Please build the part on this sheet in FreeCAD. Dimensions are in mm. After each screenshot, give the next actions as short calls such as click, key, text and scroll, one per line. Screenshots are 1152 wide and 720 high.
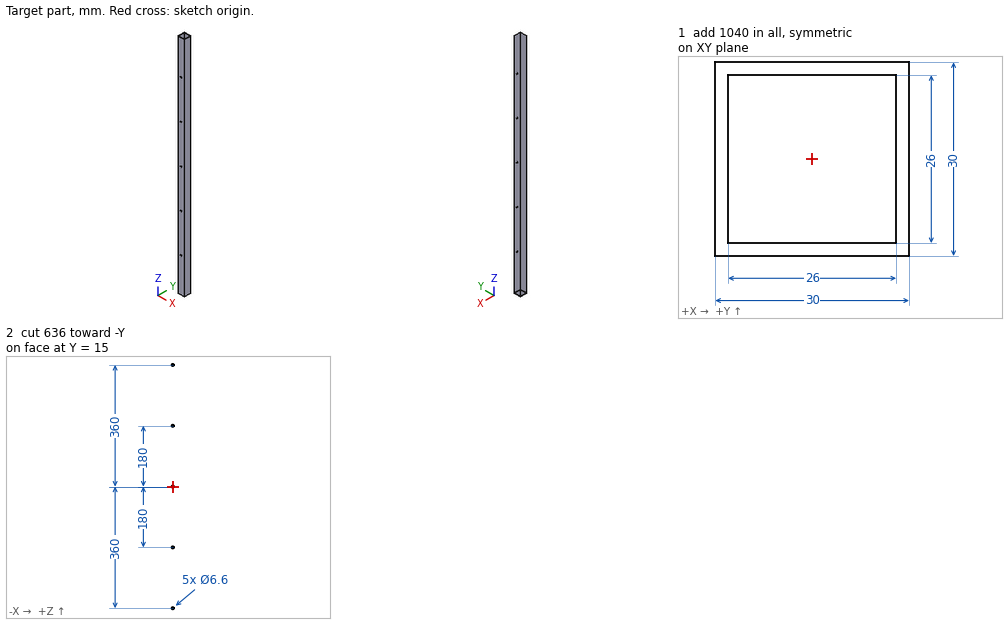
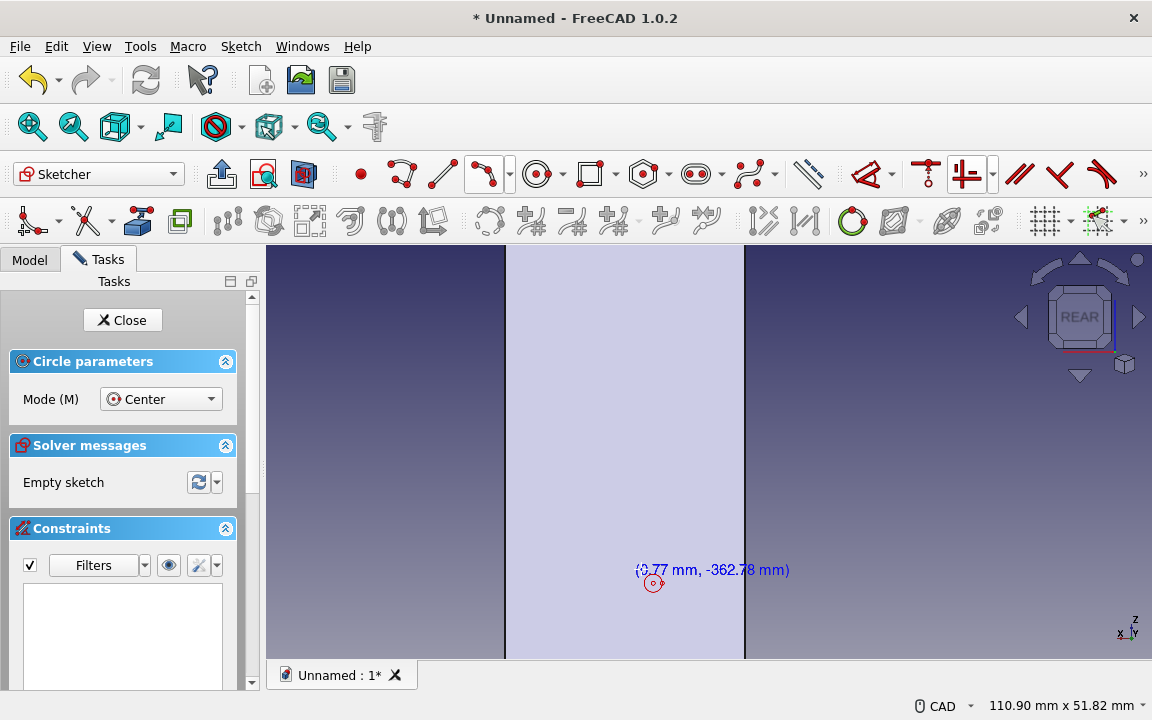
scroll(641, 597, down, 15)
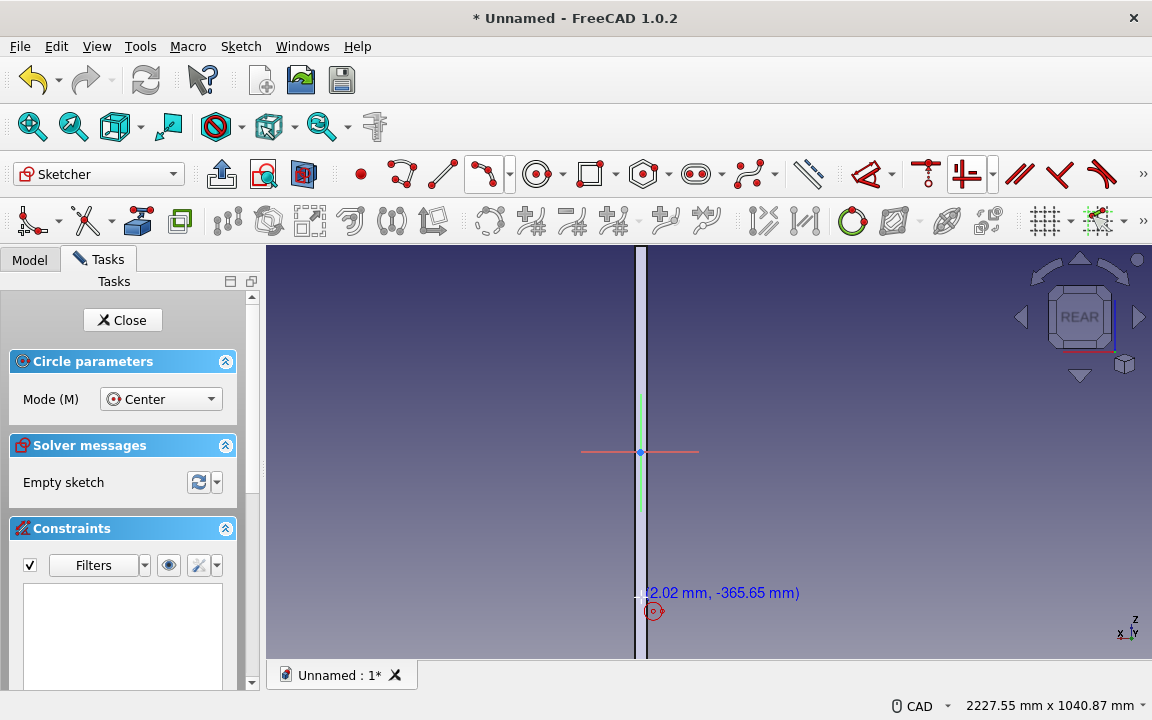
click(641, 596)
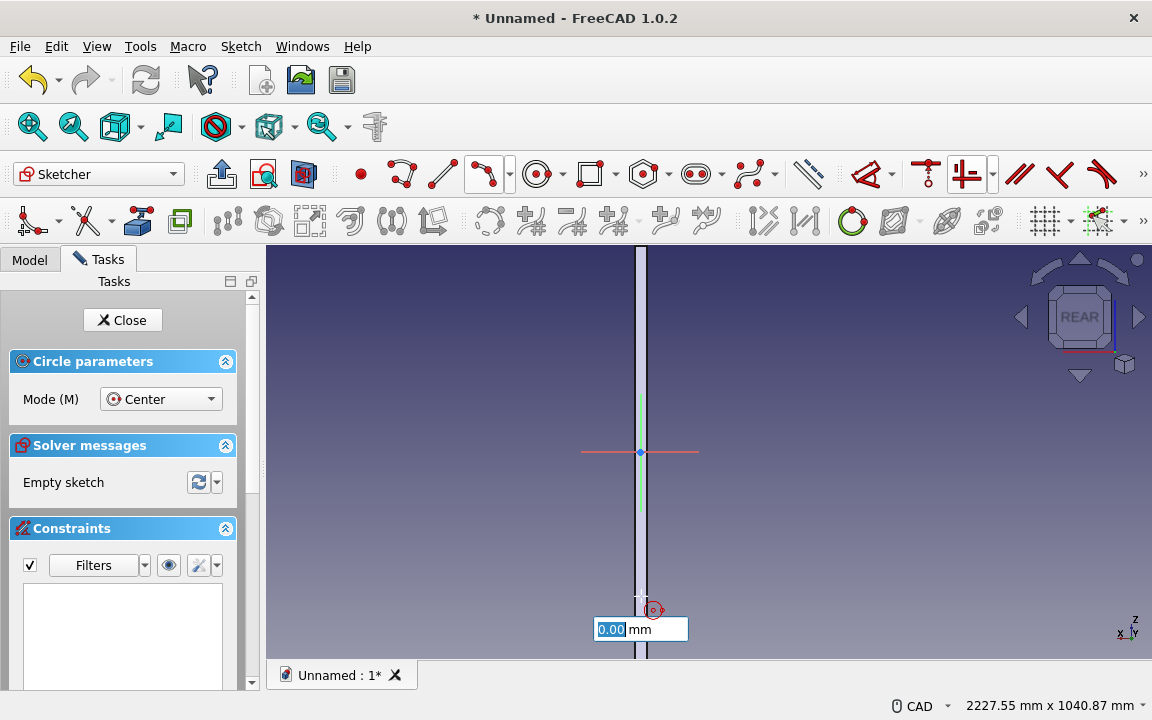
scroll(642, 595, up, 13)
move(634, 587)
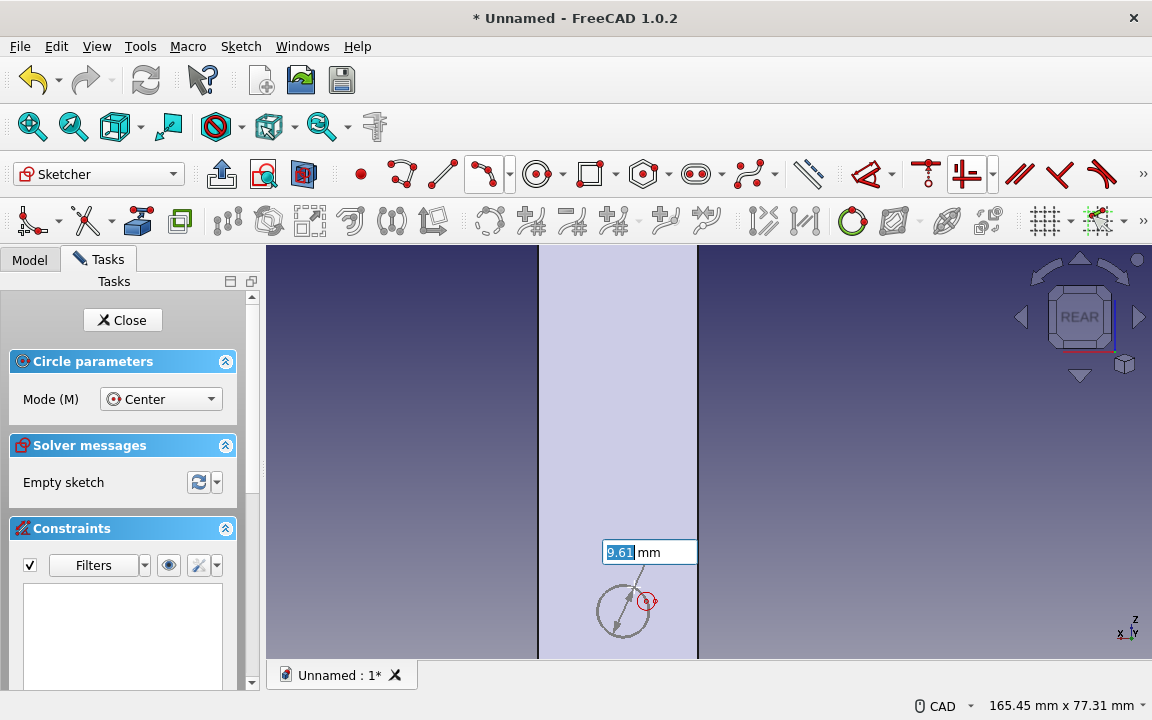
text(6.6)
key(Return)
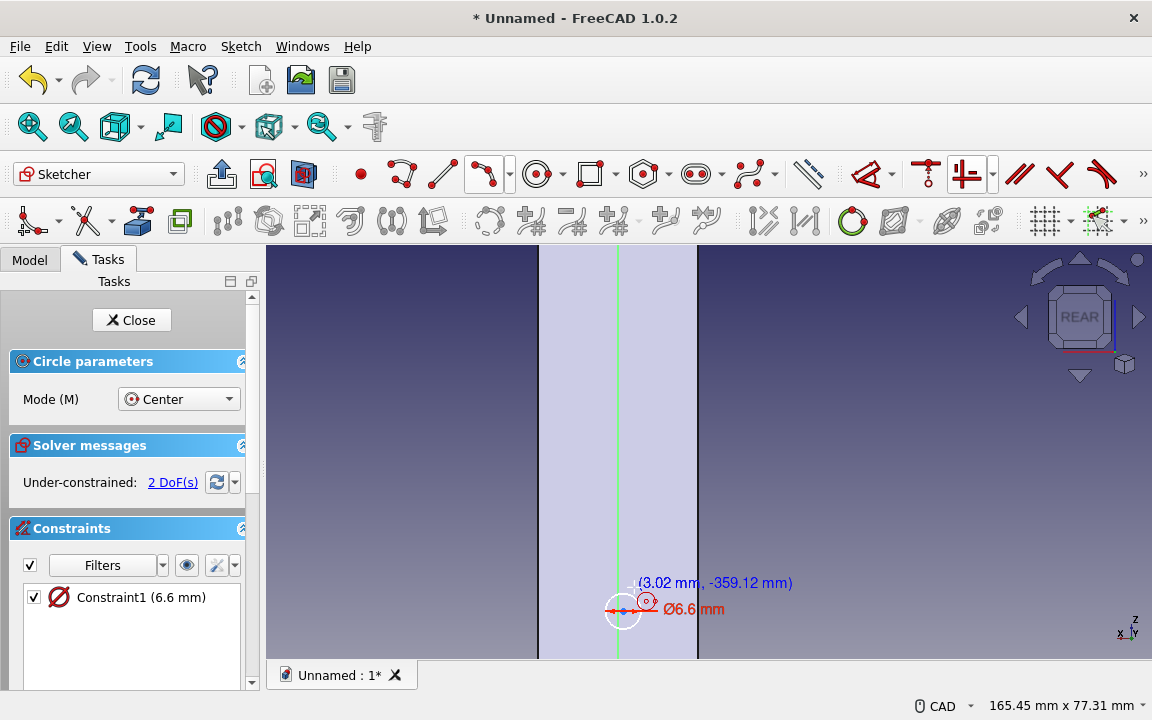
scroll(642, 568, down, 14)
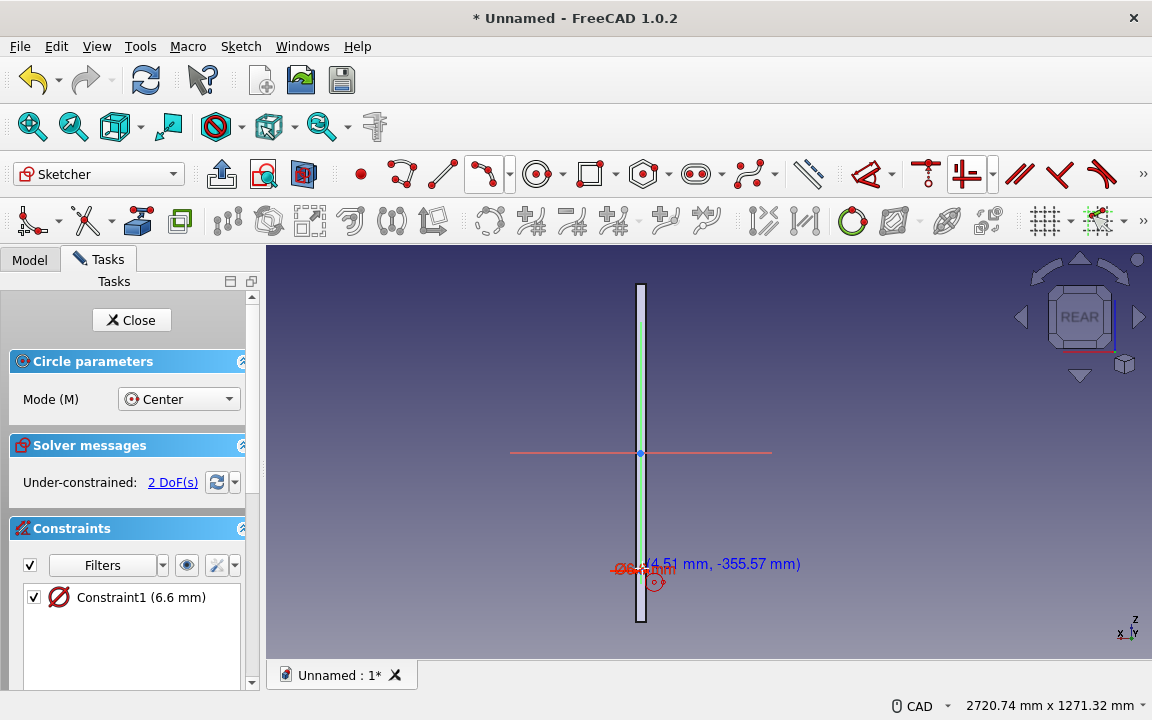
scroll(641, 512, up, 16)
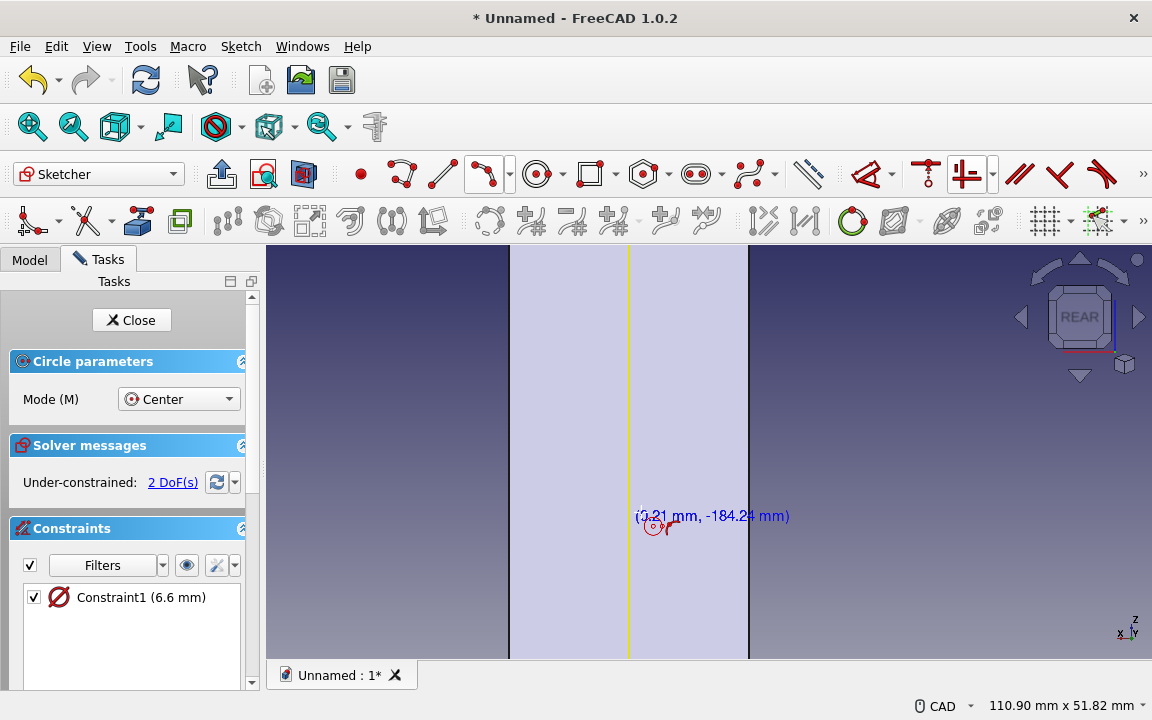
scroll(641, 525, down, 15)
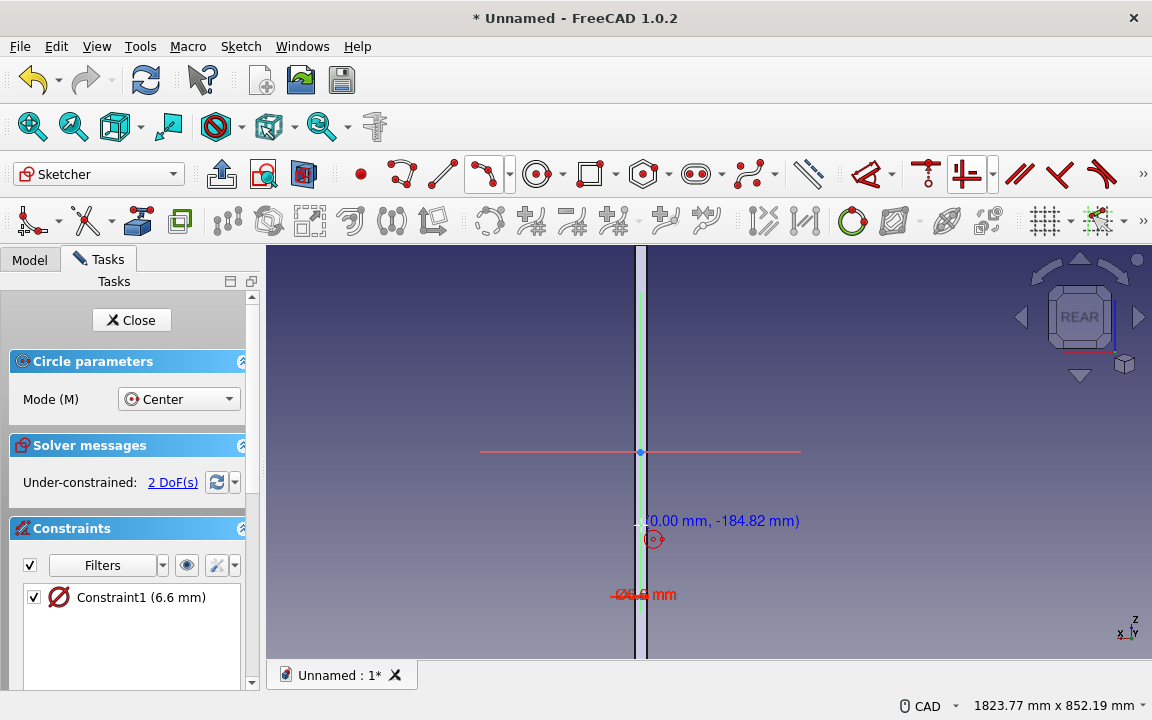
click(641, 524)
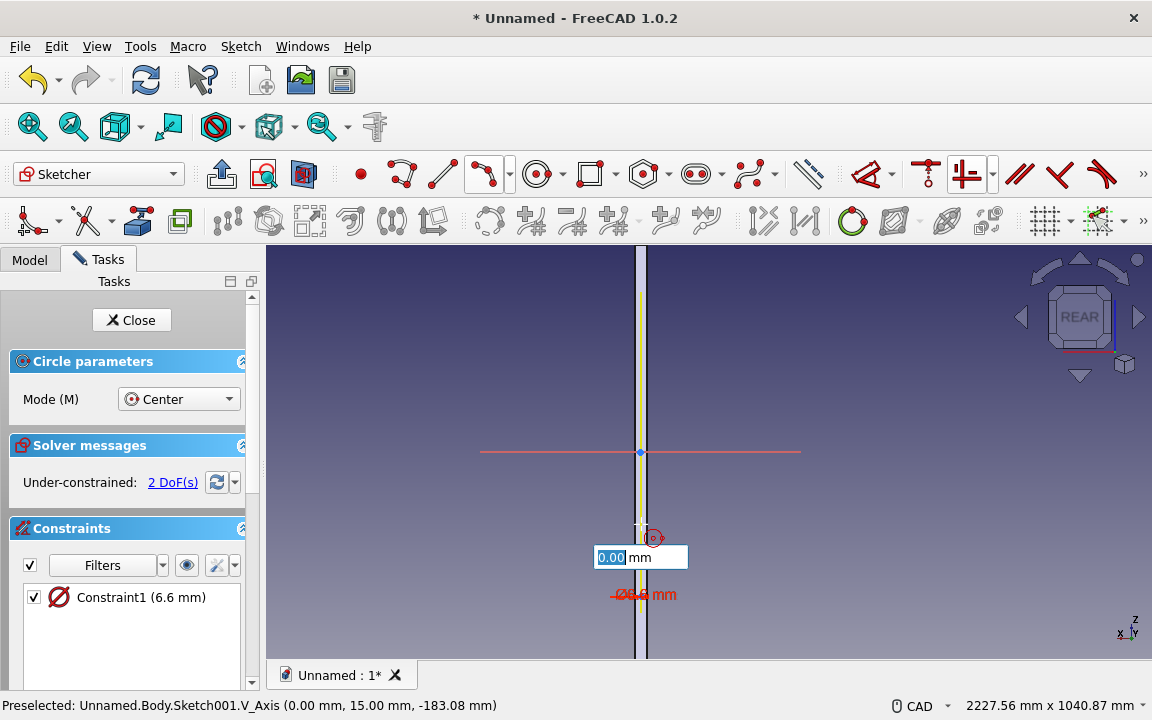
scroll(642, 523, up, 13)
move(637, 519)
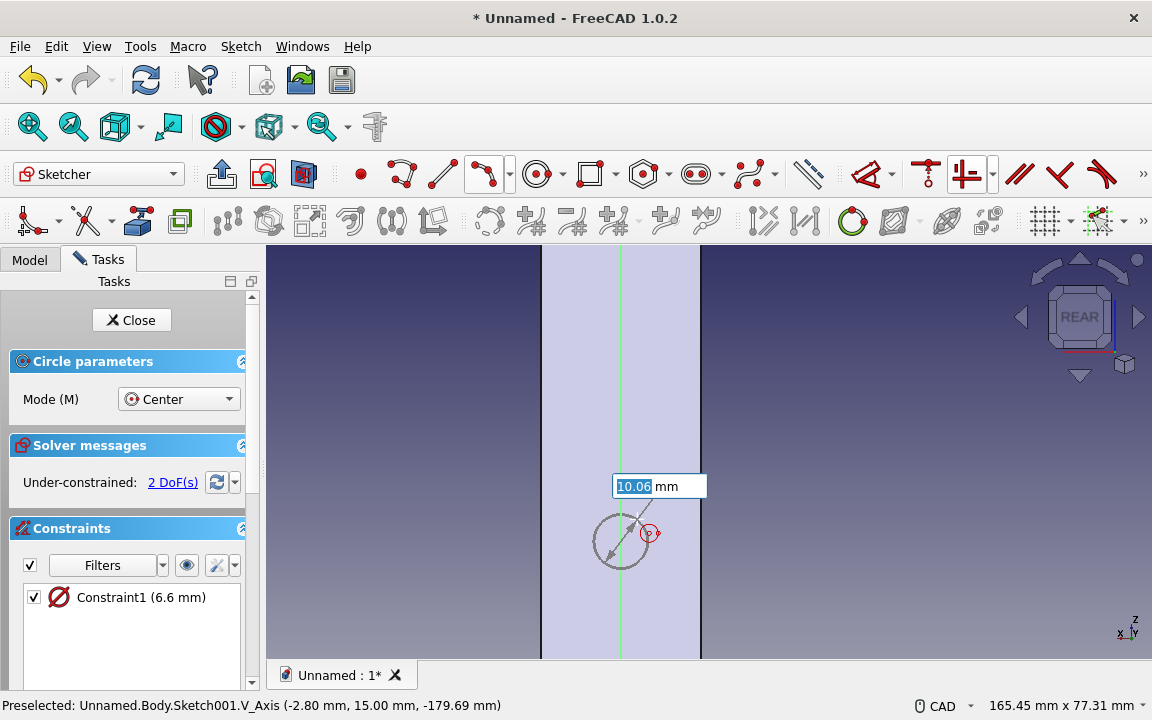
text(6.6)
key(Return)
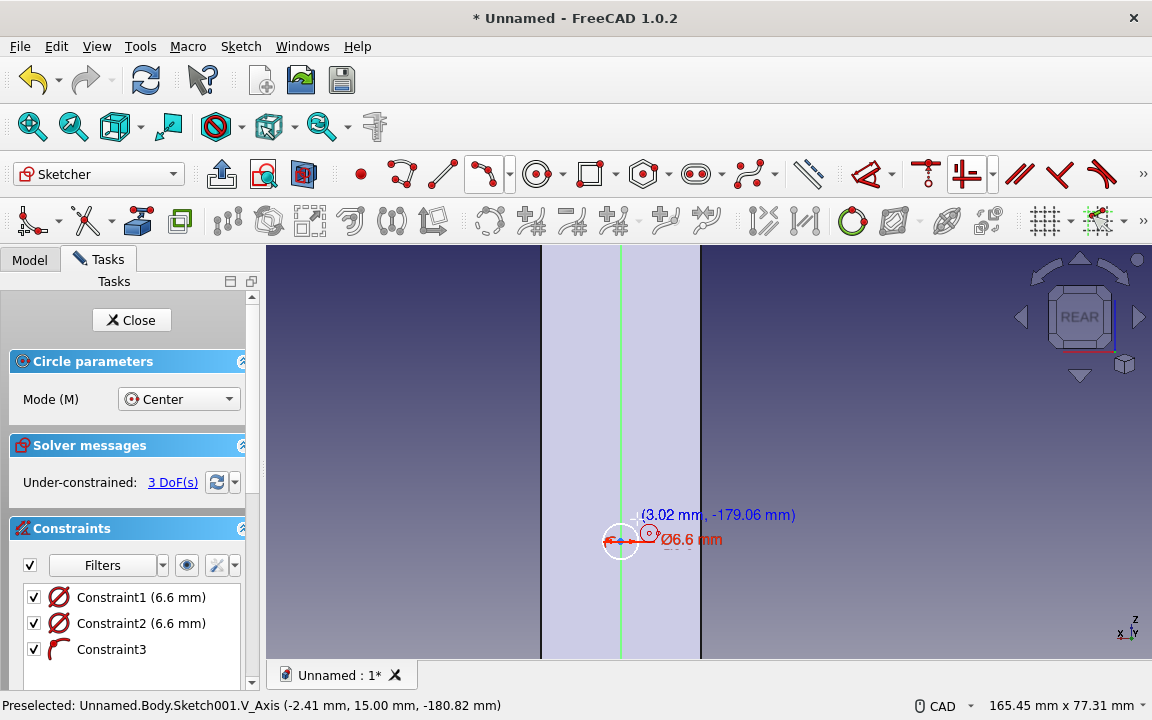
scroll(642, 510, down, 14)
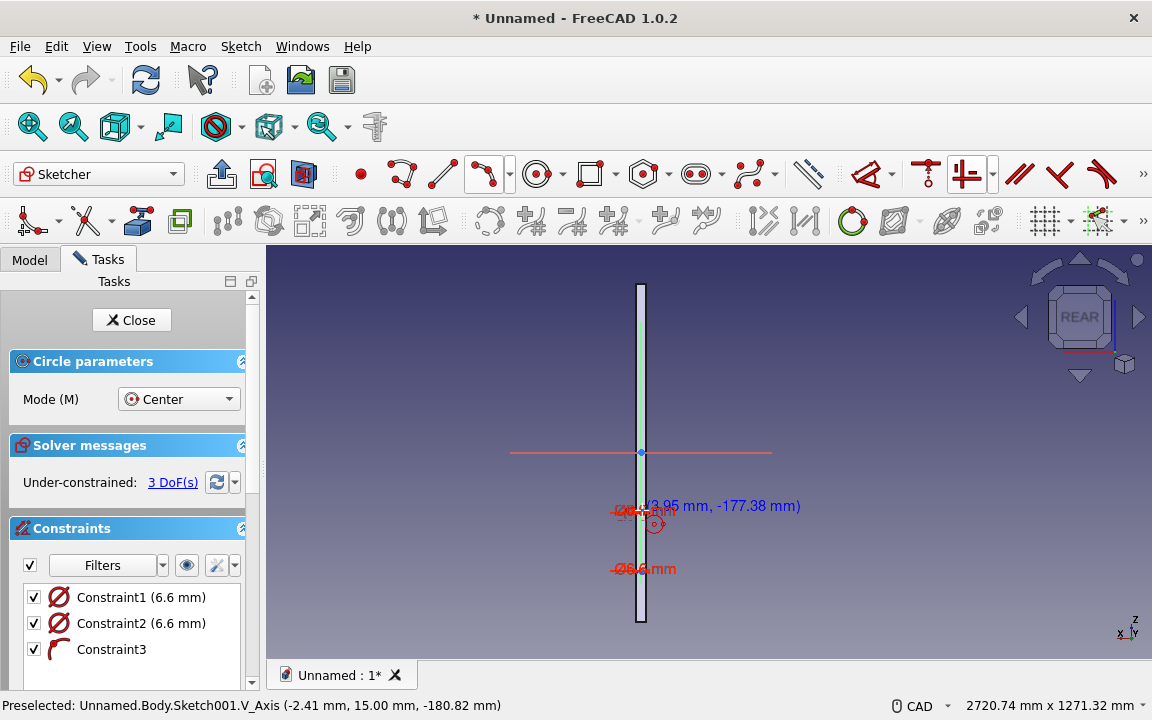
scroll(641, 453, up, 16)